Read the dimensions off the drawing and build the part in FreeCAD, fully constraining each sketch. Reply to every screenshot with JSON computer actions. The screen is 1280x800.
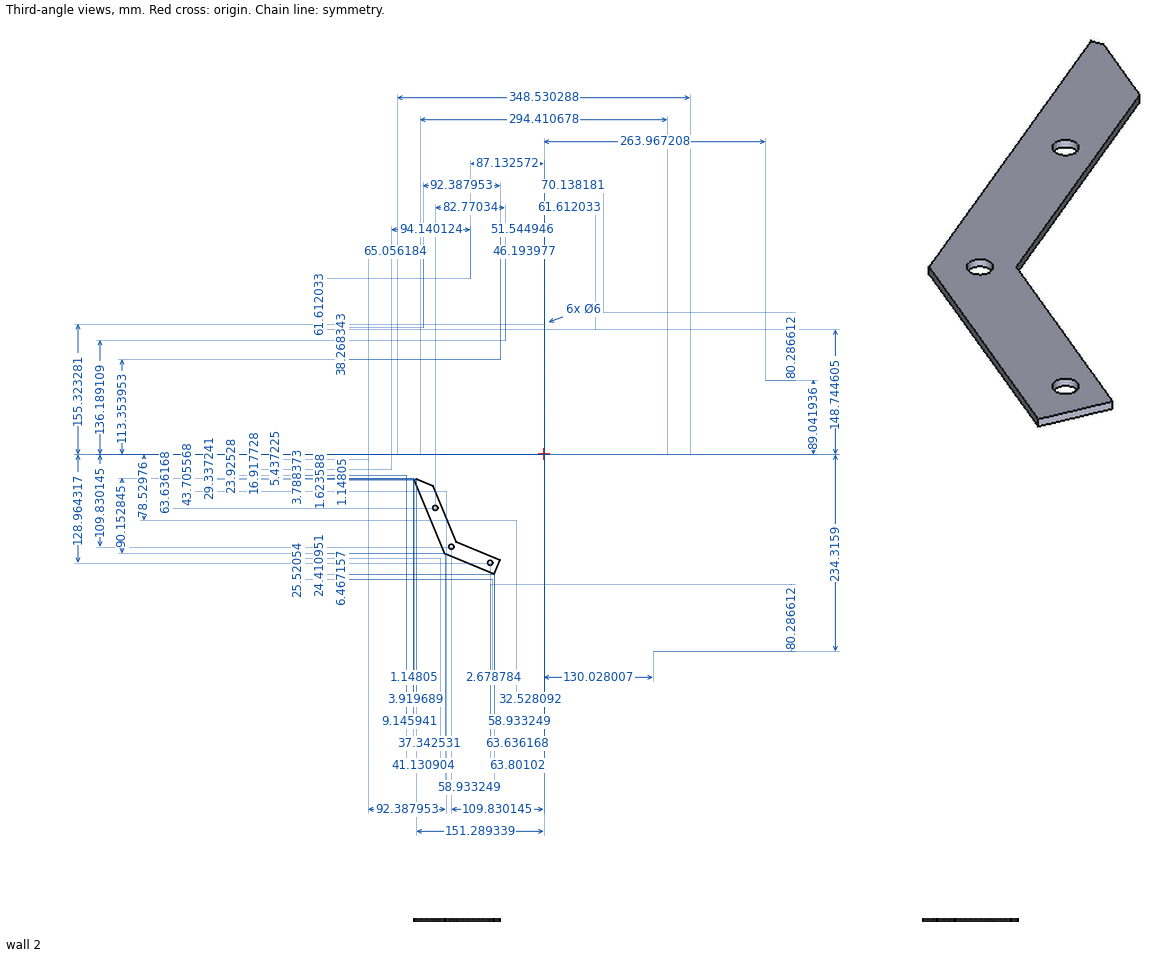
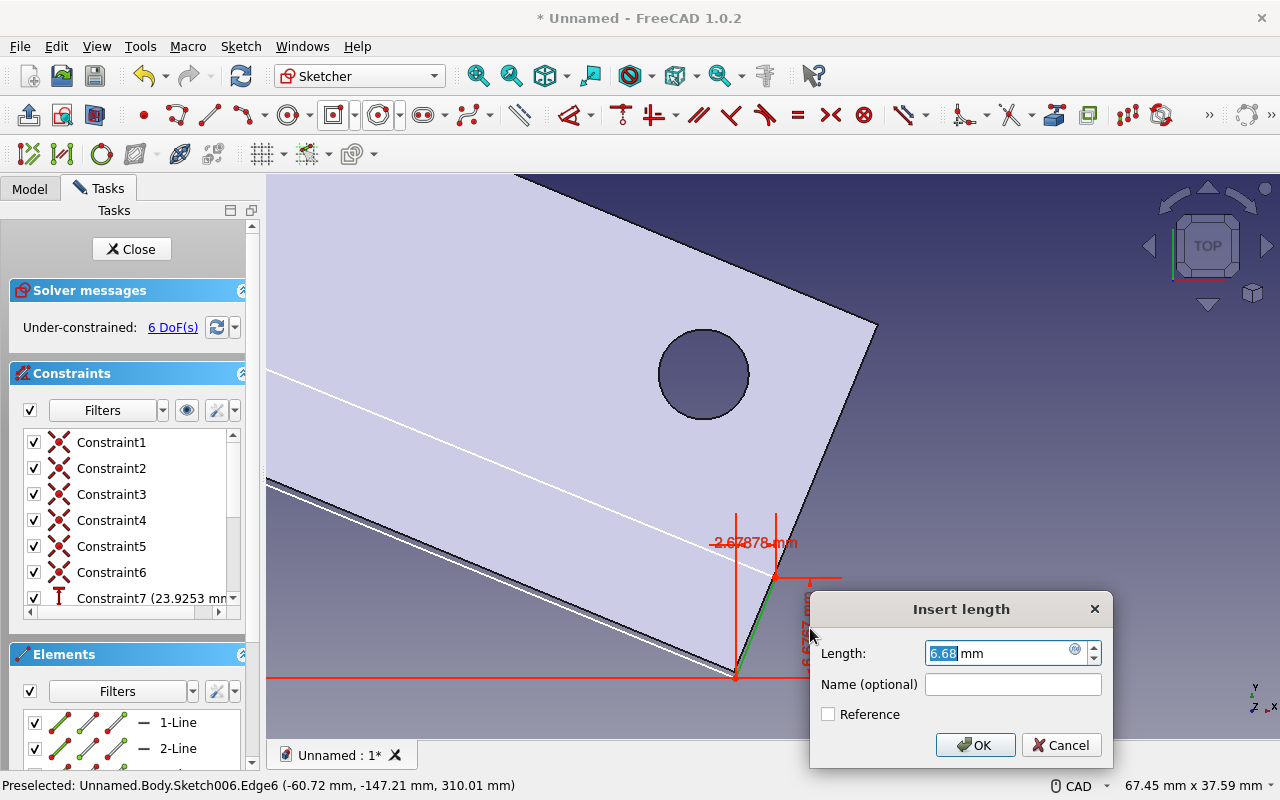
{"action": "type", "text": "6.467157"}
{"action": "key", "text": "Return"}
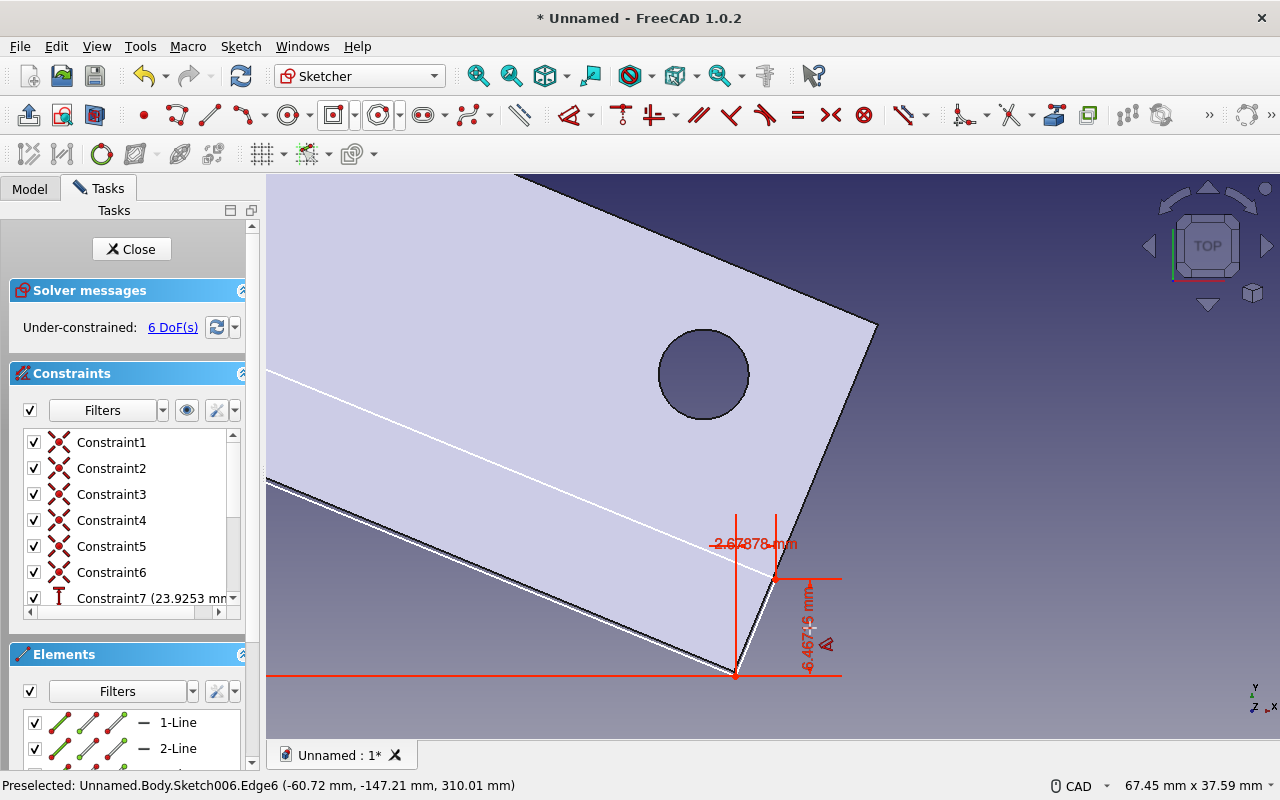
{"action": "scroll", "coordinate": [760, 635], "scroll_direction": "down", "scroll_amount": 9}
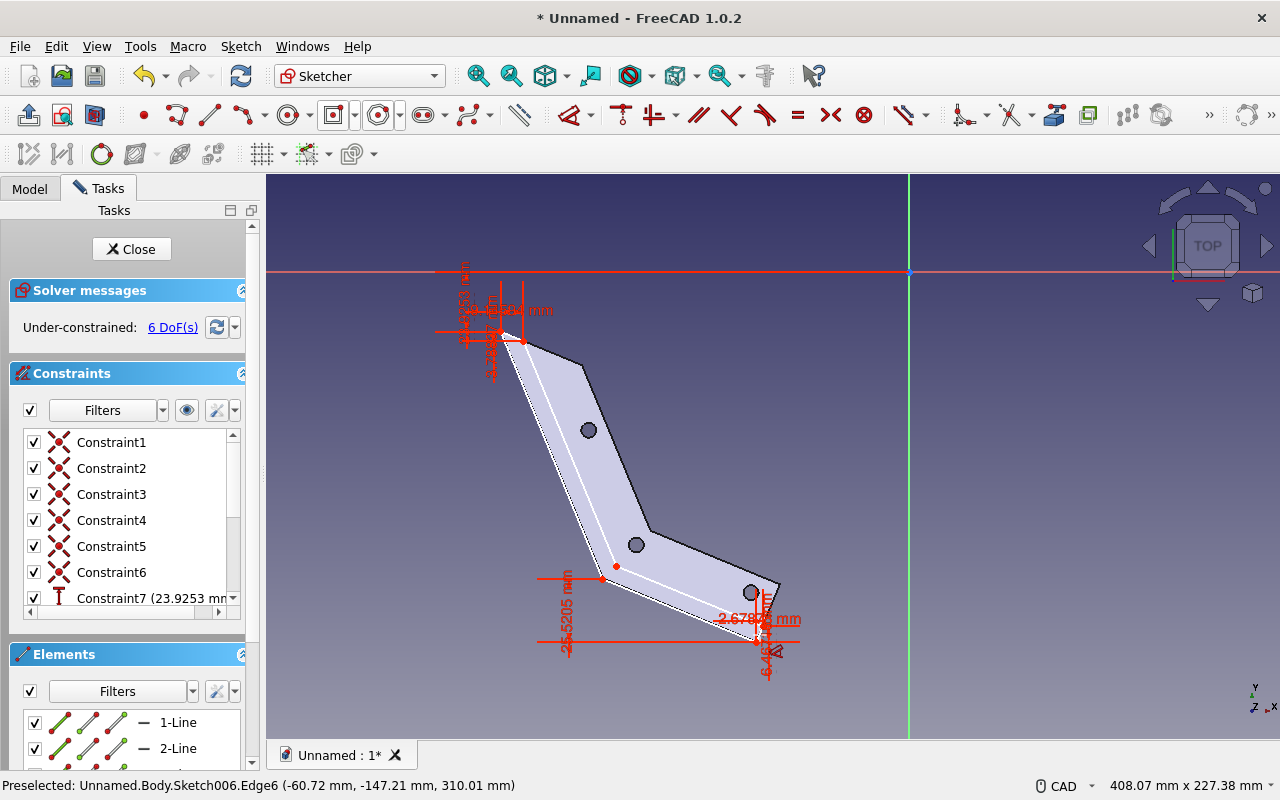
{"action": "left_click", "coordinate": [763, 626]}
{"action": "left_click", "coordinate": [836, 238]}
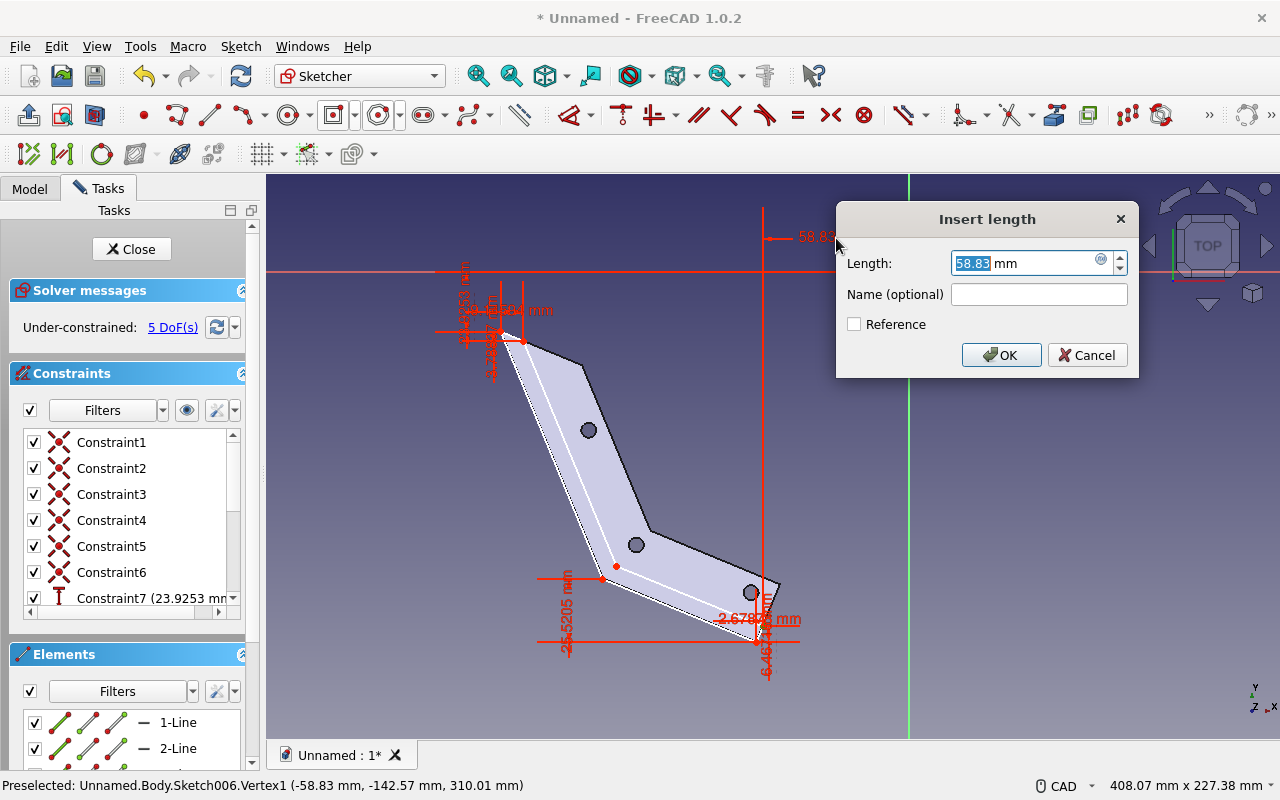
{"action": "type", "text": "58.933249"}
{"action": "key", "text": "Return"}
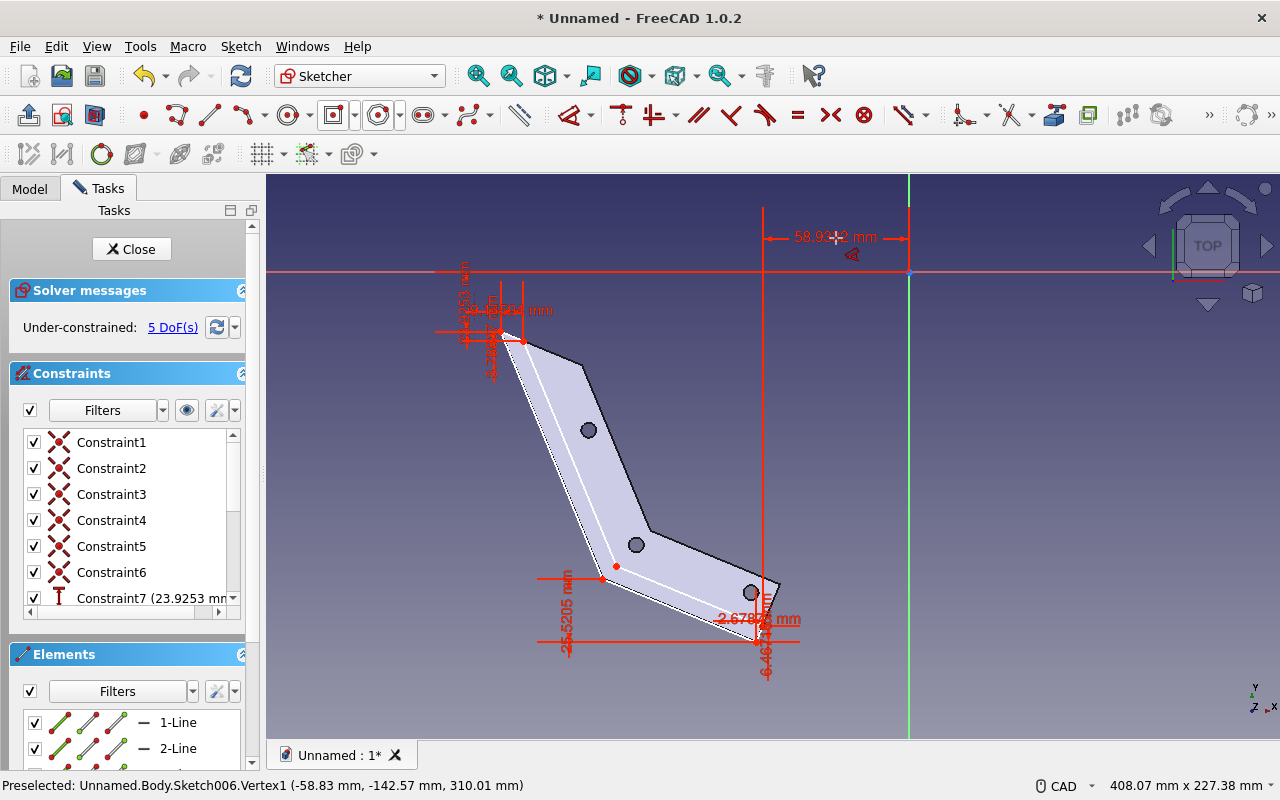
{"action": "left_click", "coordinate": [719, 608]}
{"action": "left_click", "coordinate": [690, 660]}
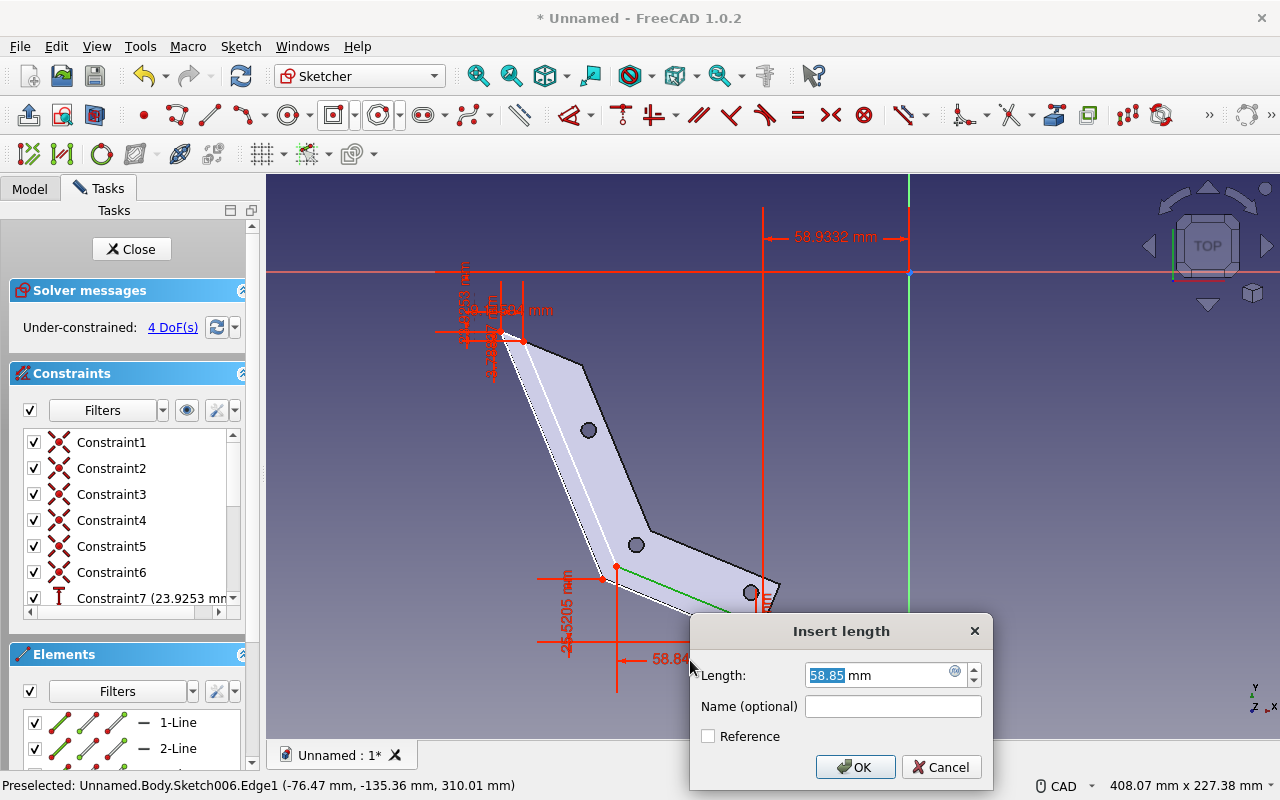
{"action": "type", "text": "58.933249"}
{"action": "key", "text": "Return"}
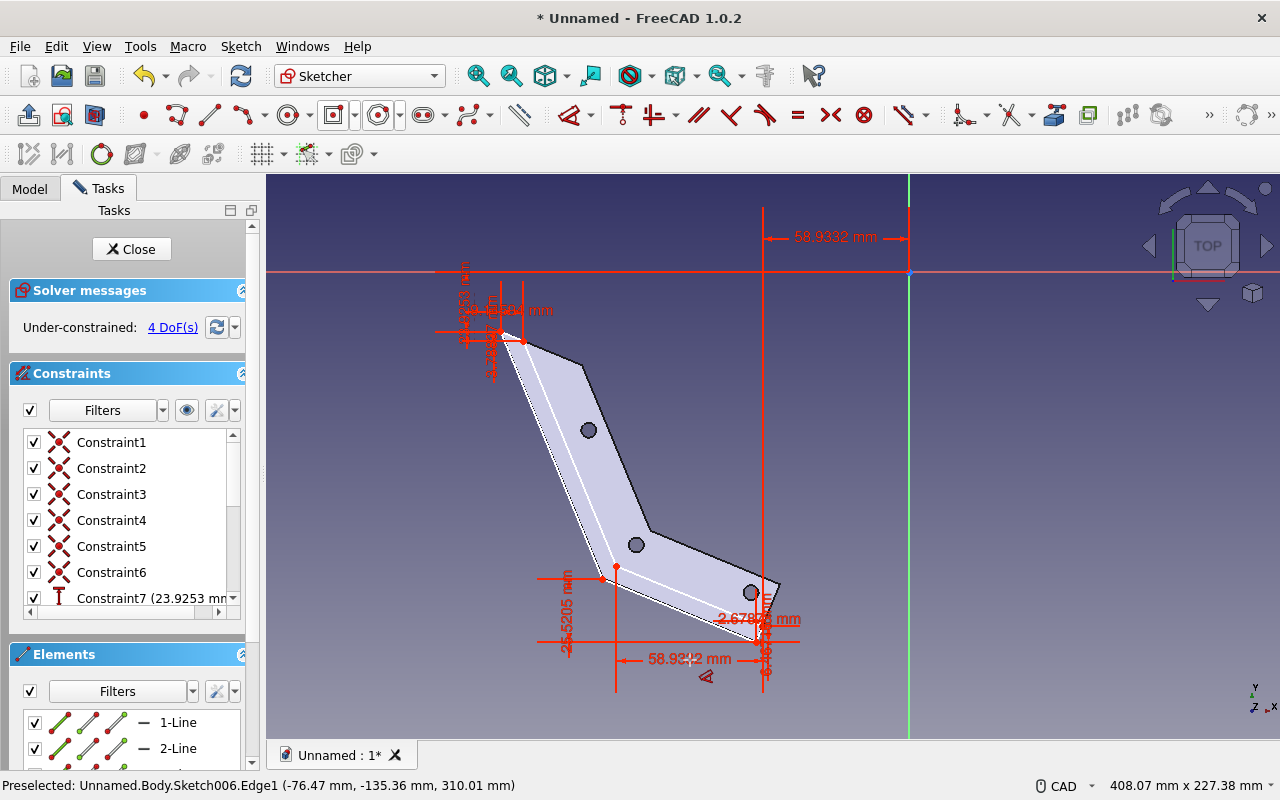
{"action": "left_click", "coordinate": [719, 608]}
{"action": "left_click", "coordinate": [582, 582]}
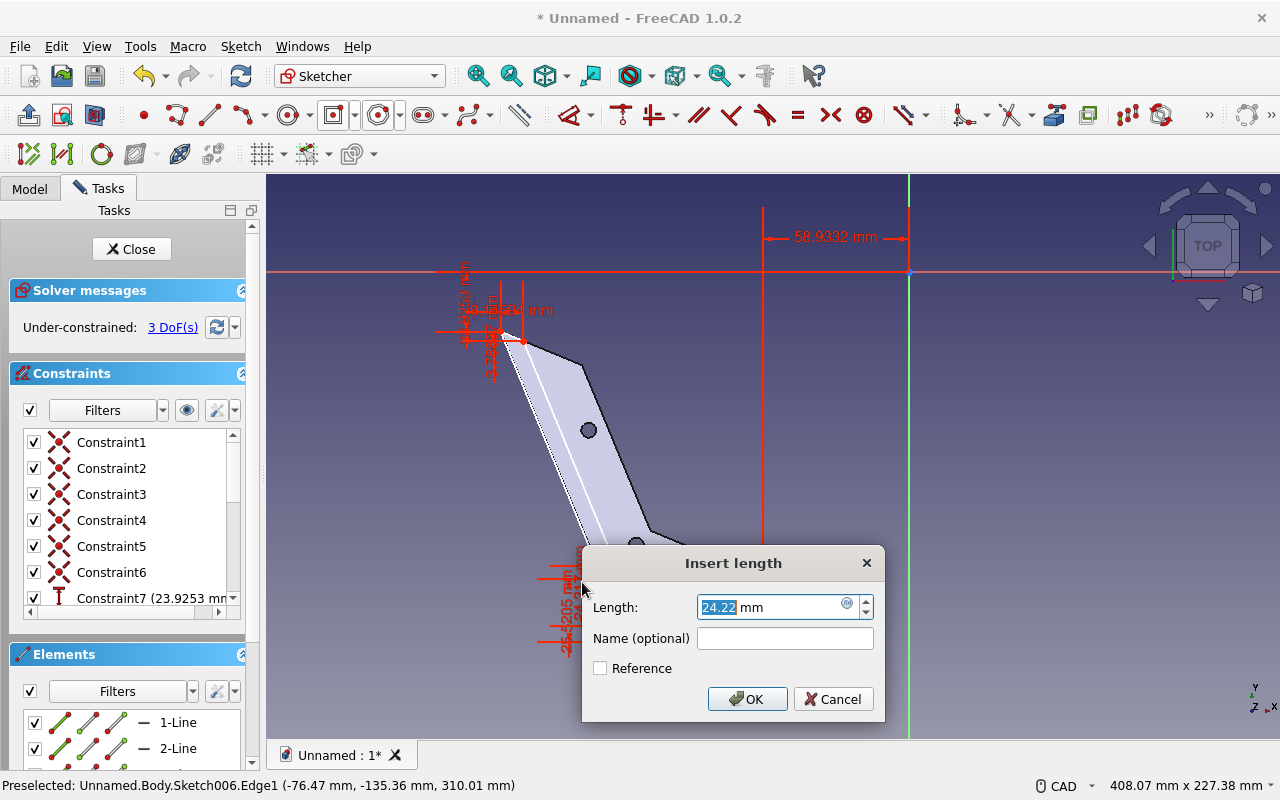
{"action": "type", "text": "24.410951"}
{"action": "key", "text": "Return"}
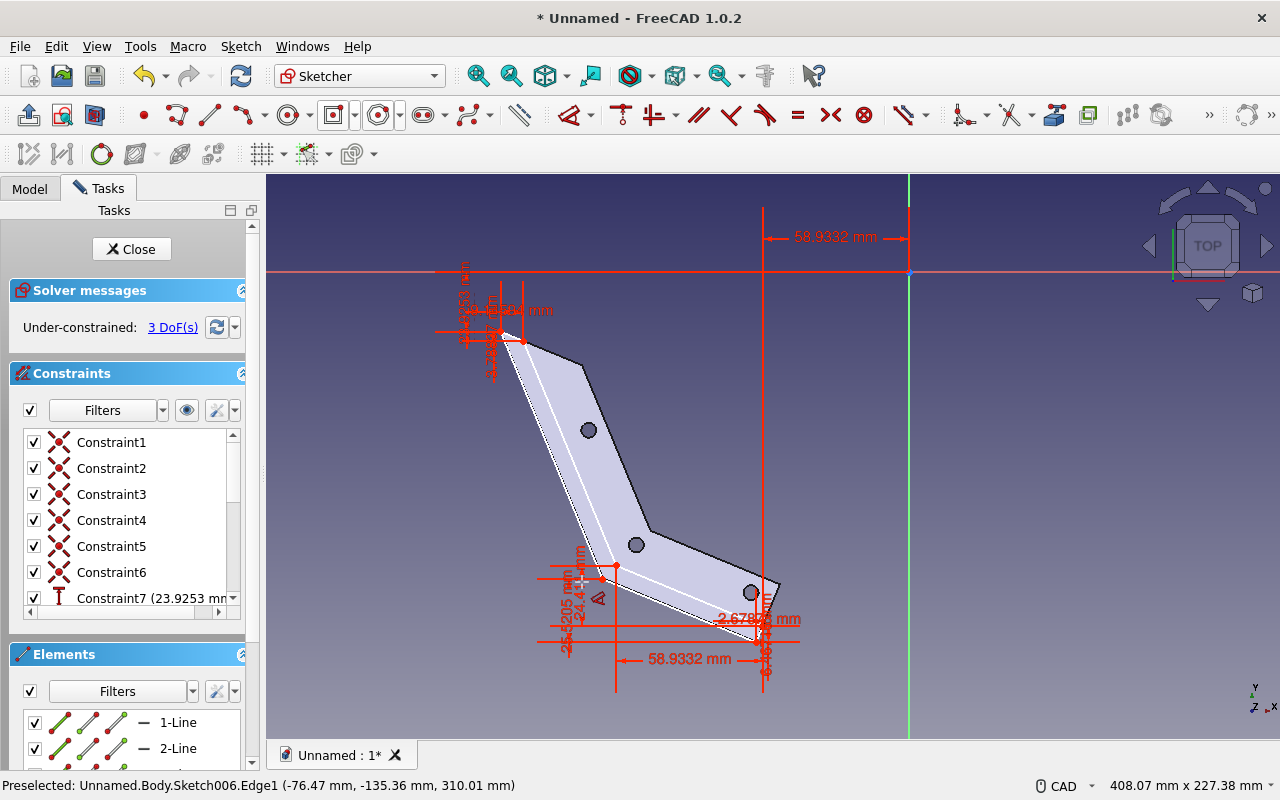
{"action": "left_click", "coordinate": [588, 498]}
{"action": "left_click", "coordinate": [591, 307]}